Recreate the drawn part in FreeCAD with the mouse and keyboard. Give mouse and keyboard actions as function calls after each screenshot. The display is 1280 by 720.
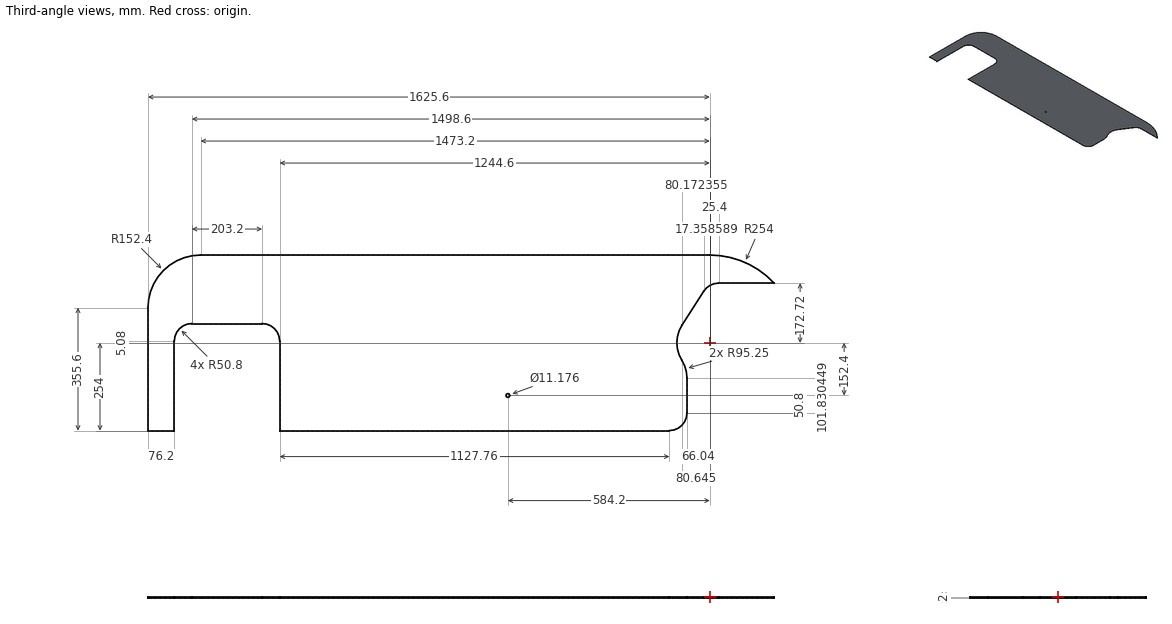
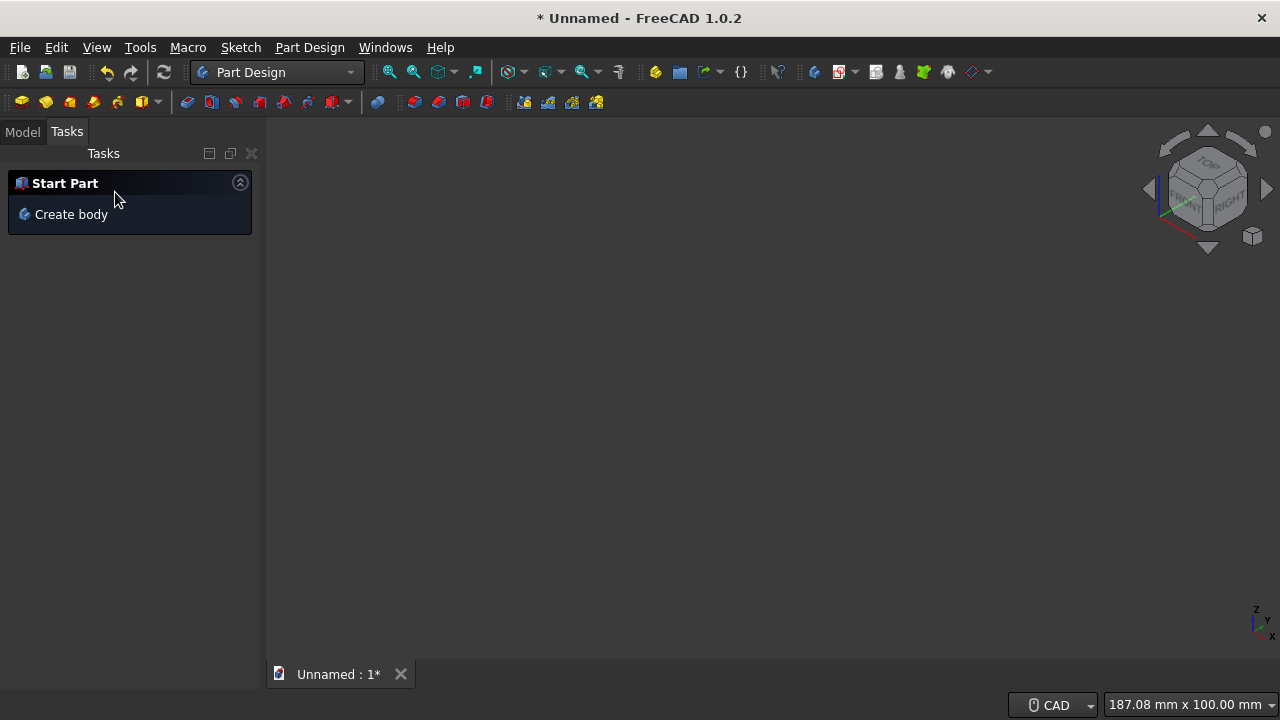
click(390, 72)